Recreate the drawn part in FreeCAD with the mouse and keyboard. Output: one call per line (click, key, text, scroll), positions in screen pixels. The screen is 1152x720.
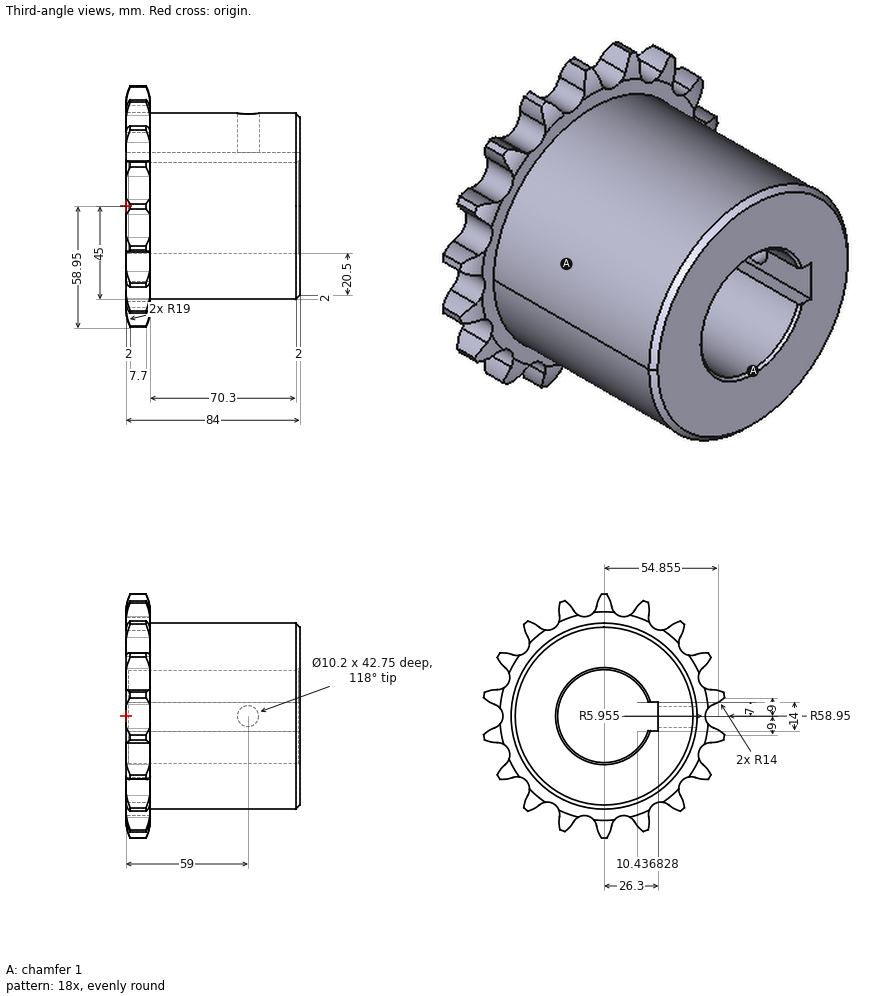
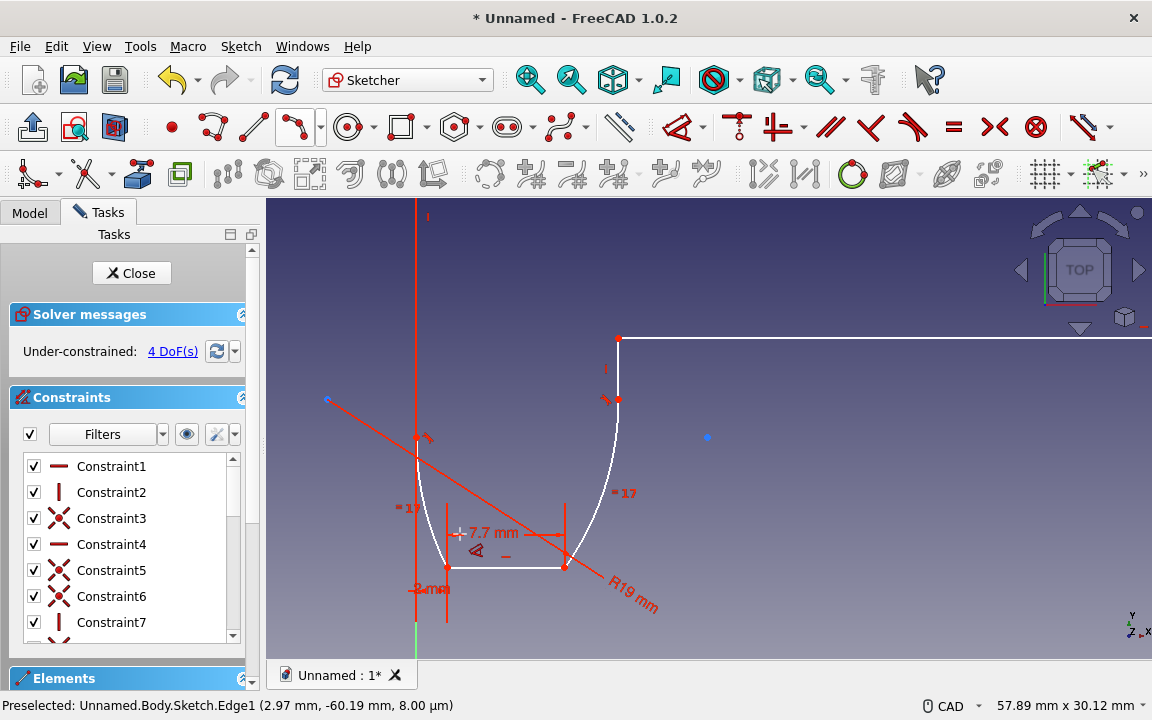
click(618, 338)
click(382, 282)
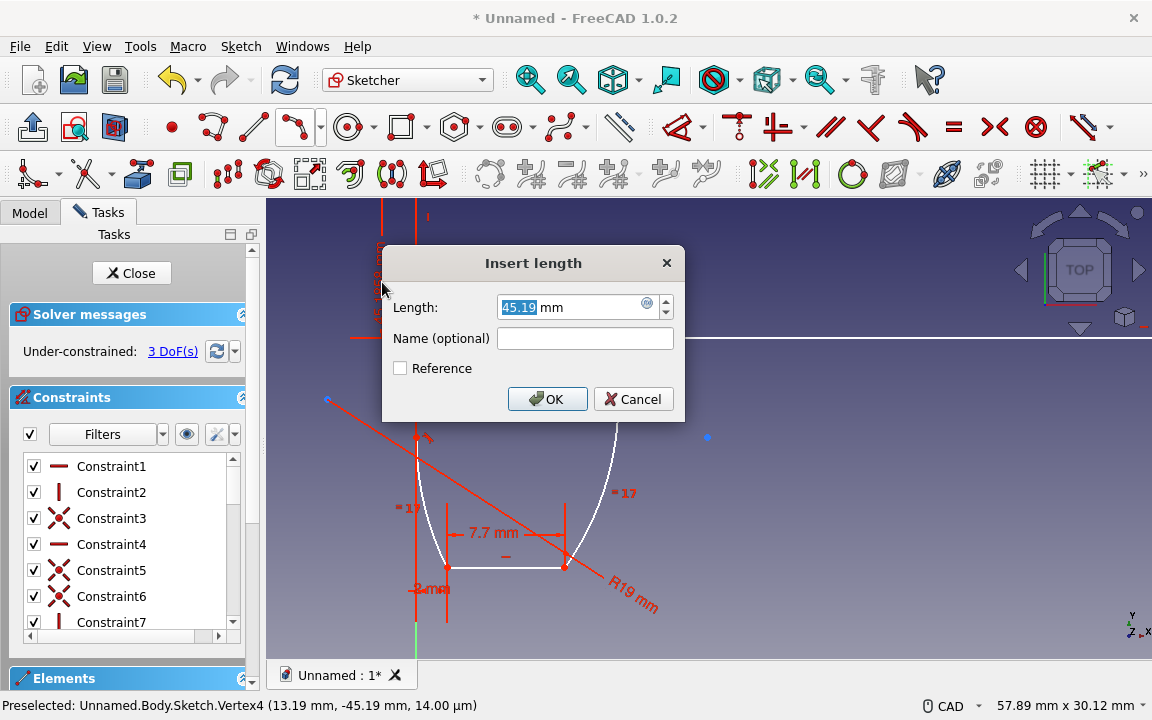
text(45)
key(Return)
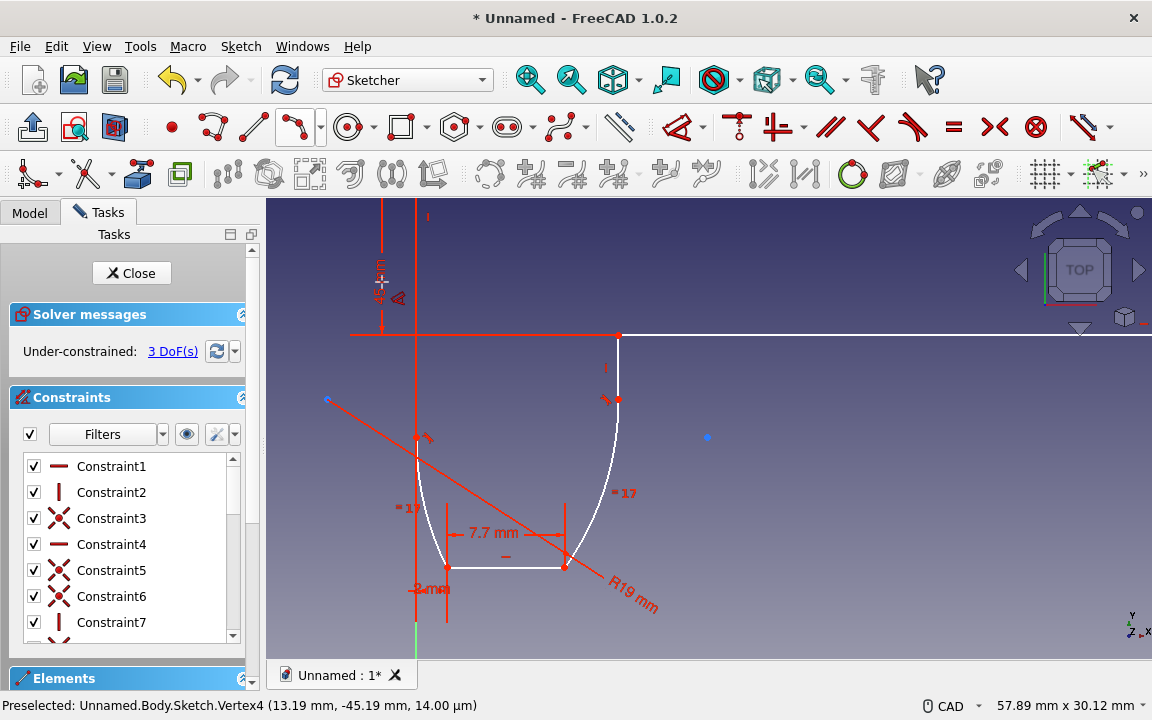
click(934, 335)
click(803, 369)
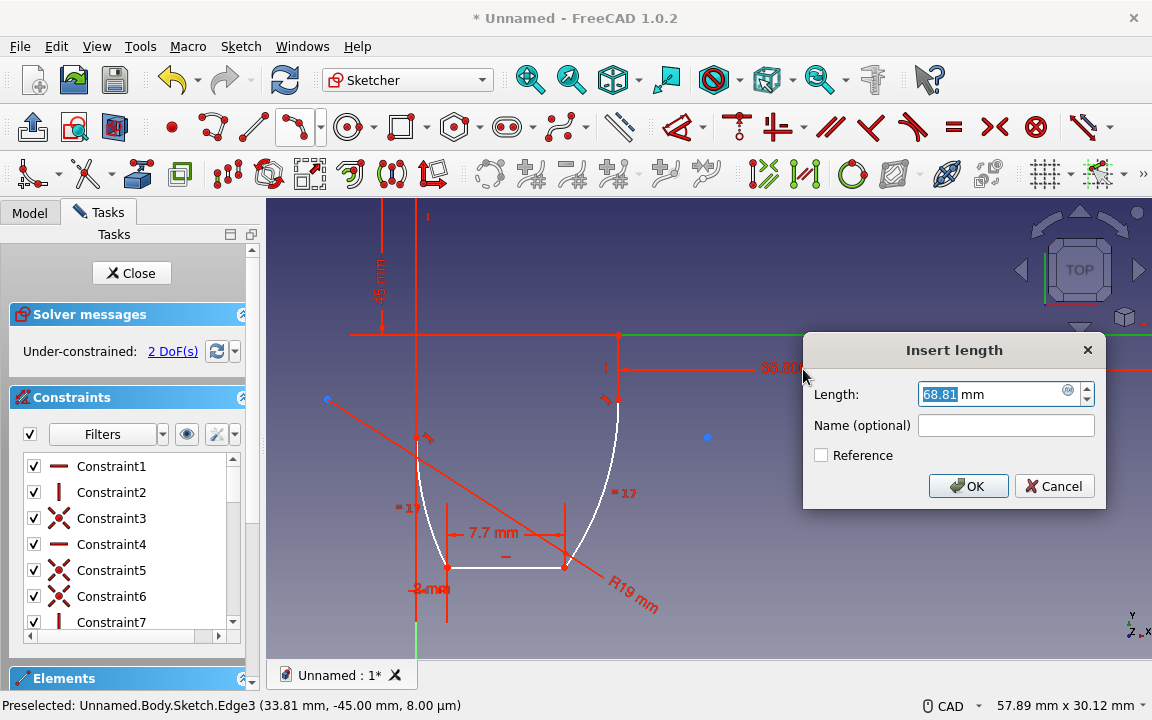
text(70.3)
key(Return)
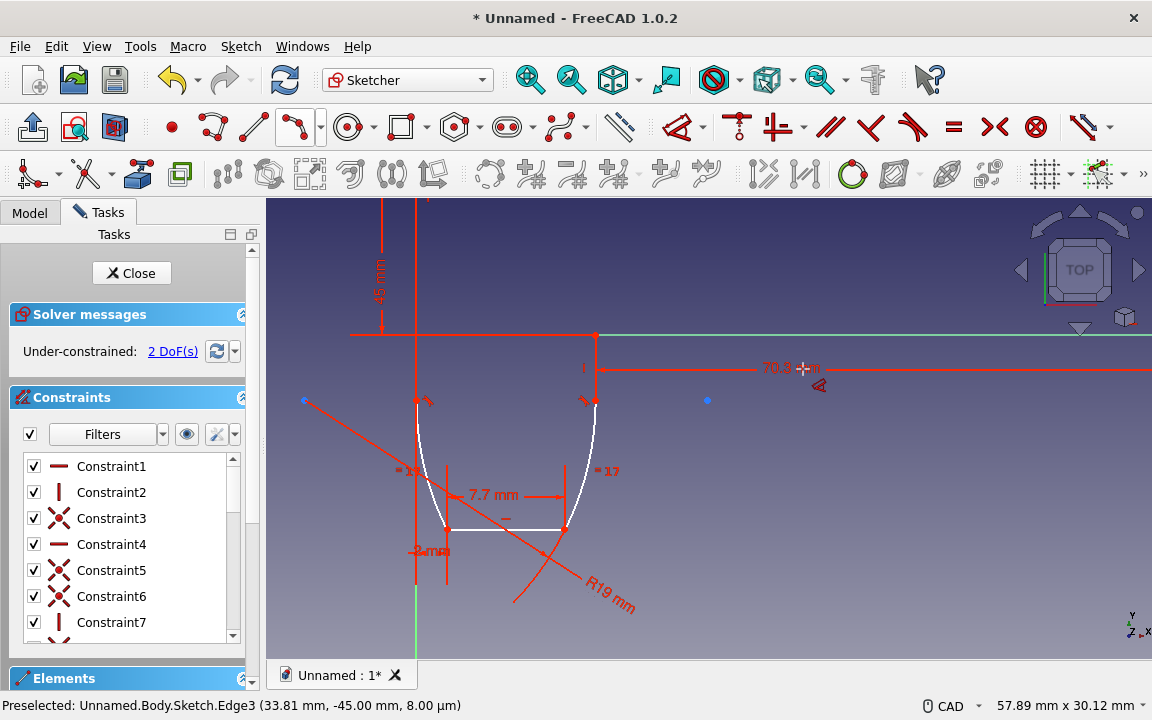
scroll(460, 571, down, 6)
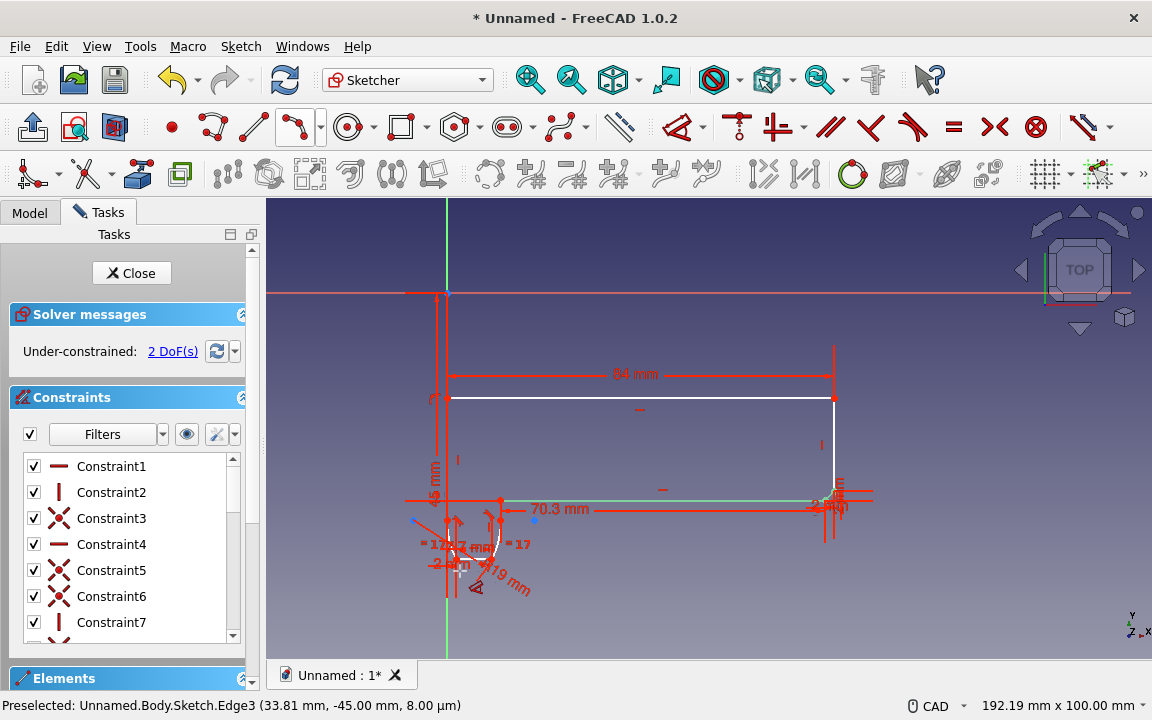
click(834, 463)
click(868, 445)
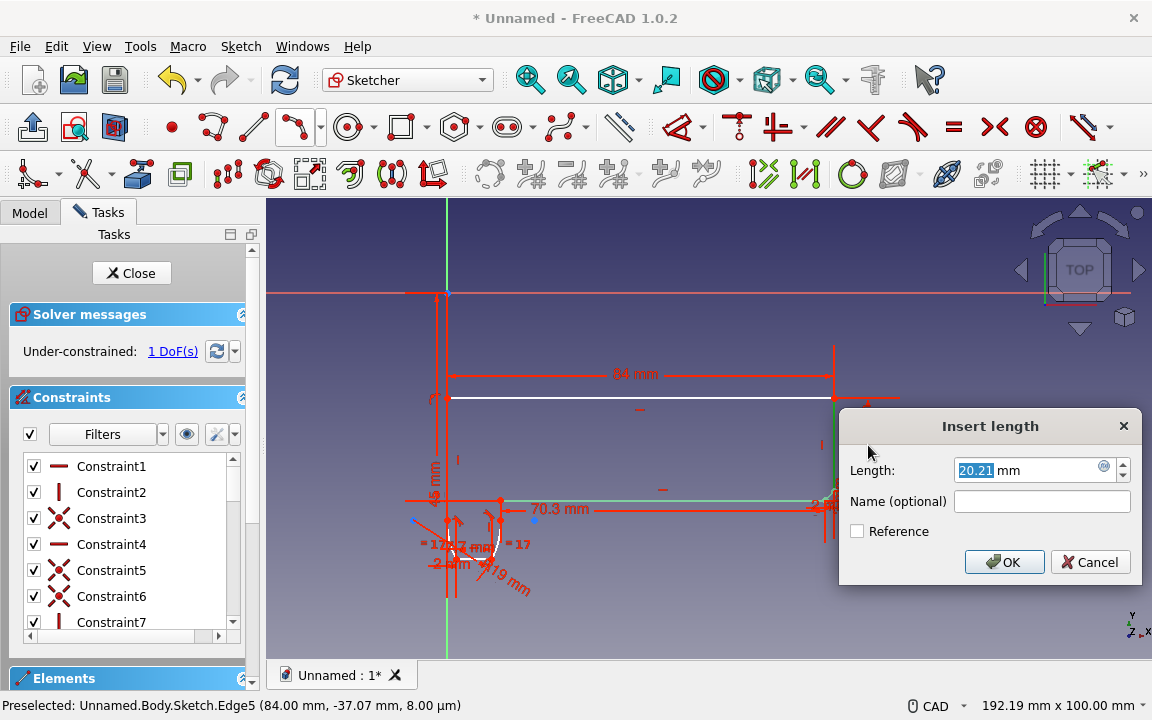
text(20.5)
key(Return)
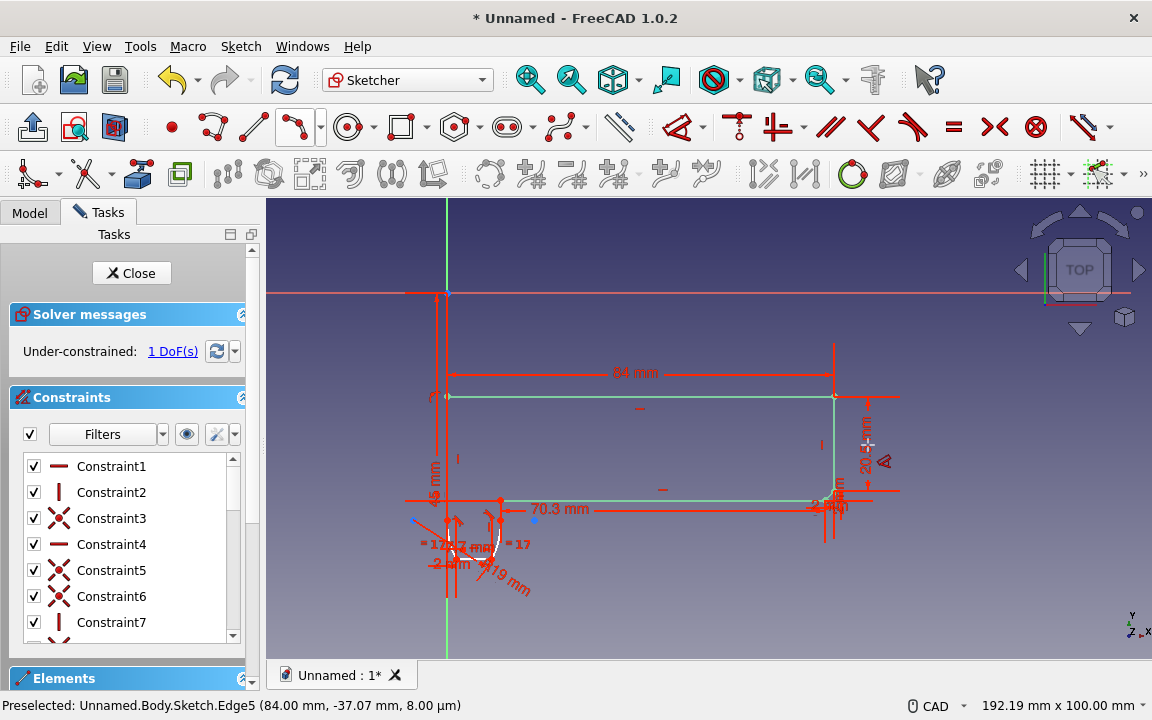
click(456, 559)
click(413, 426)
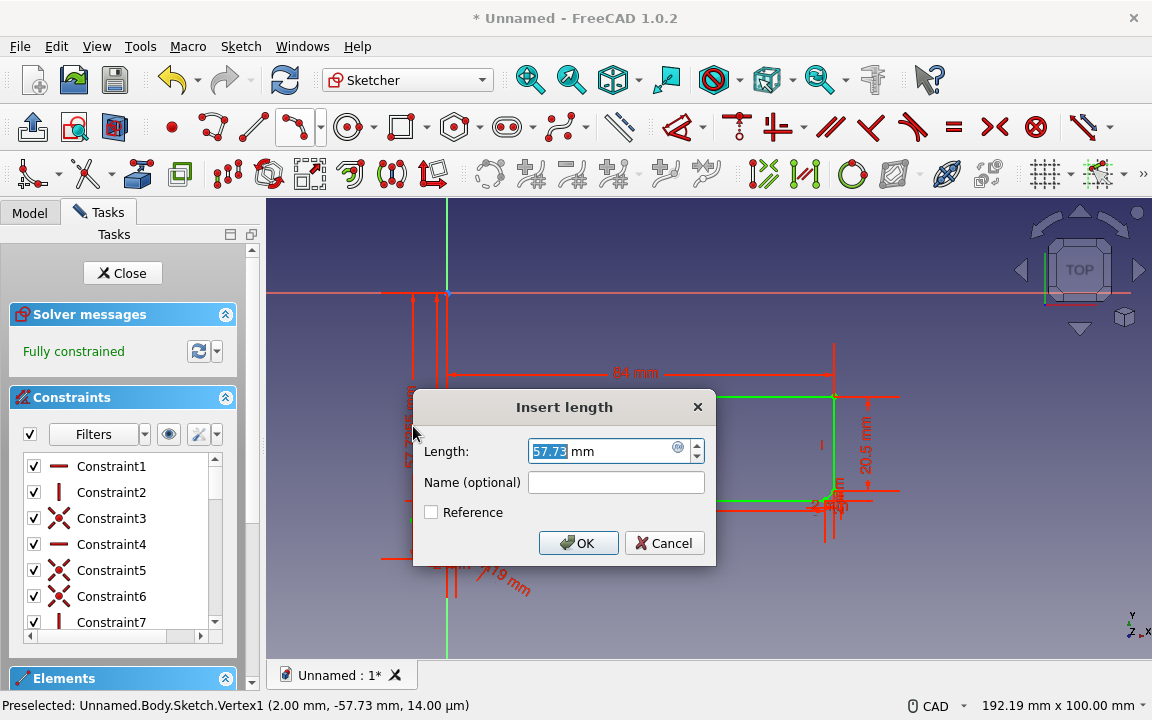
text(58.95)
key(Return)
key(Escape)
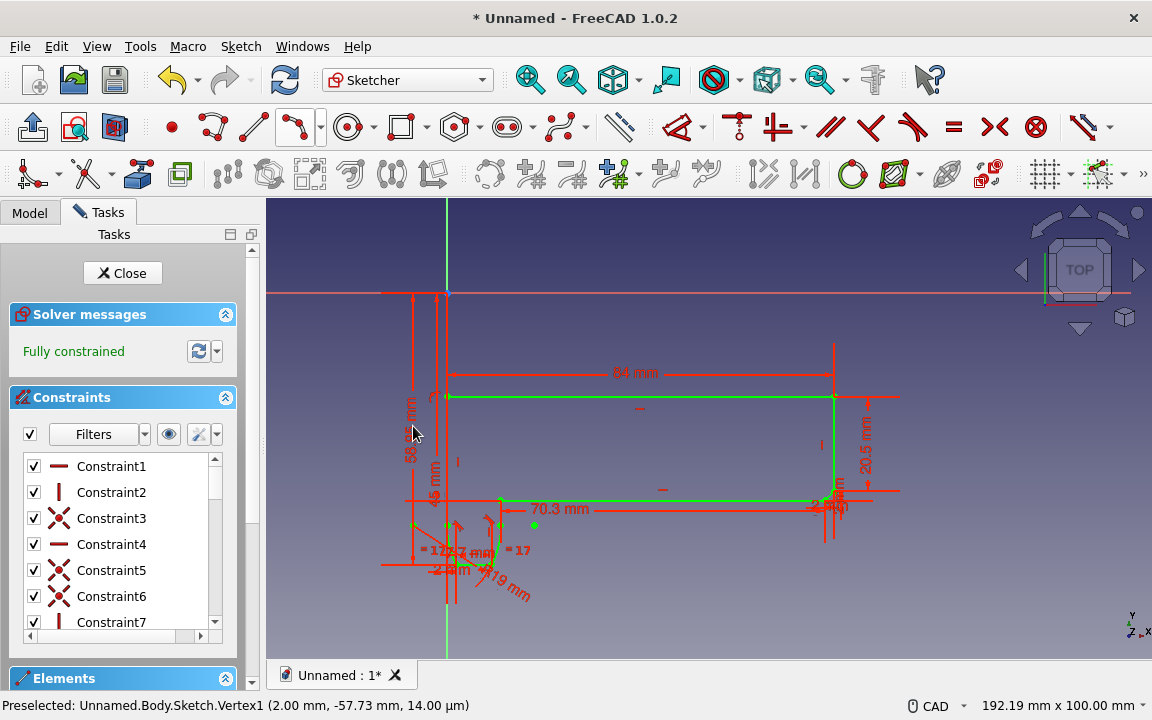
click(123, 273)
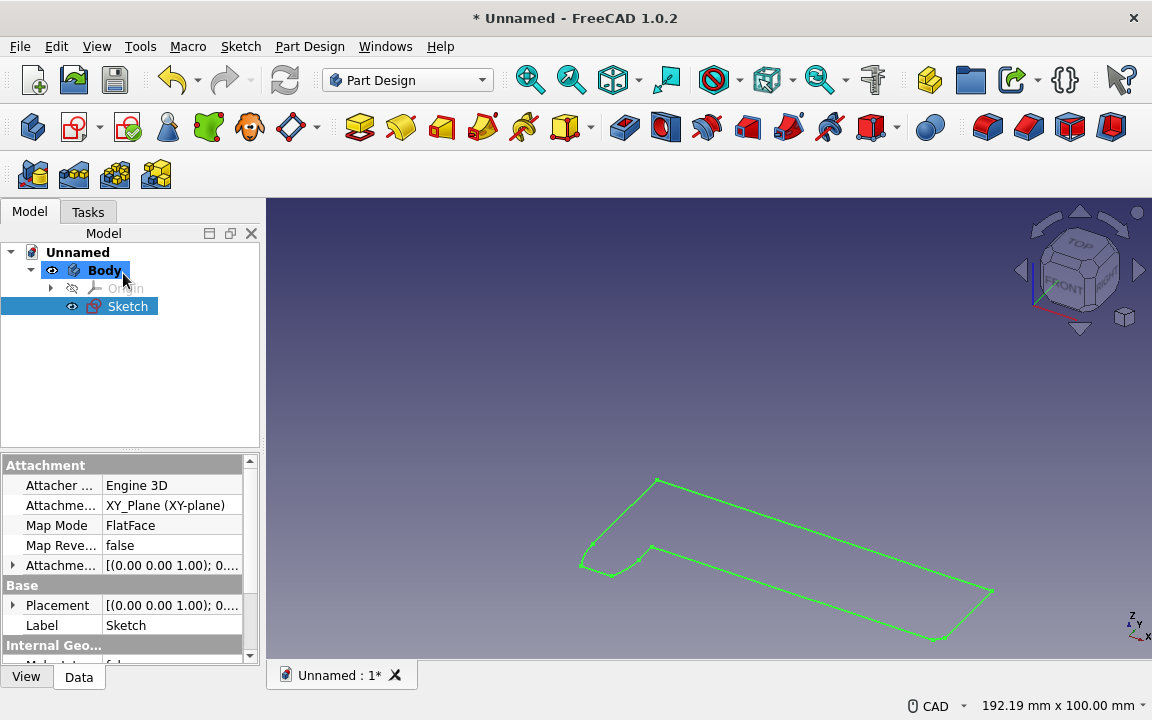
click(401, 128)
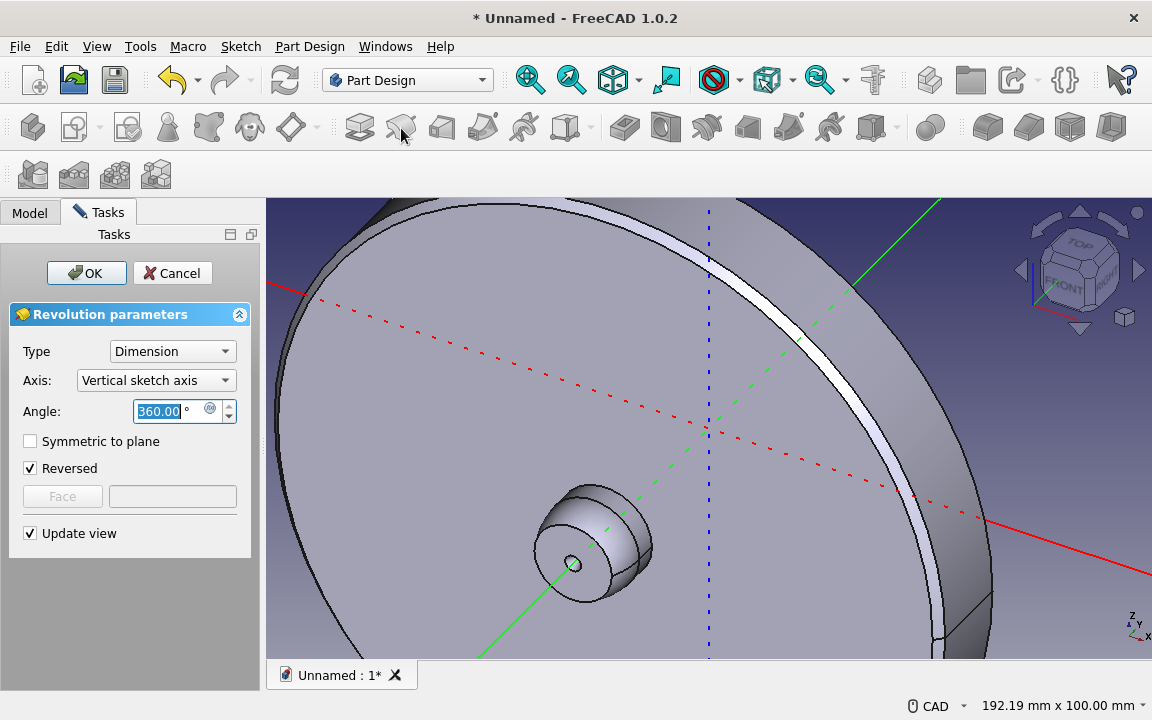
click(157, 380)